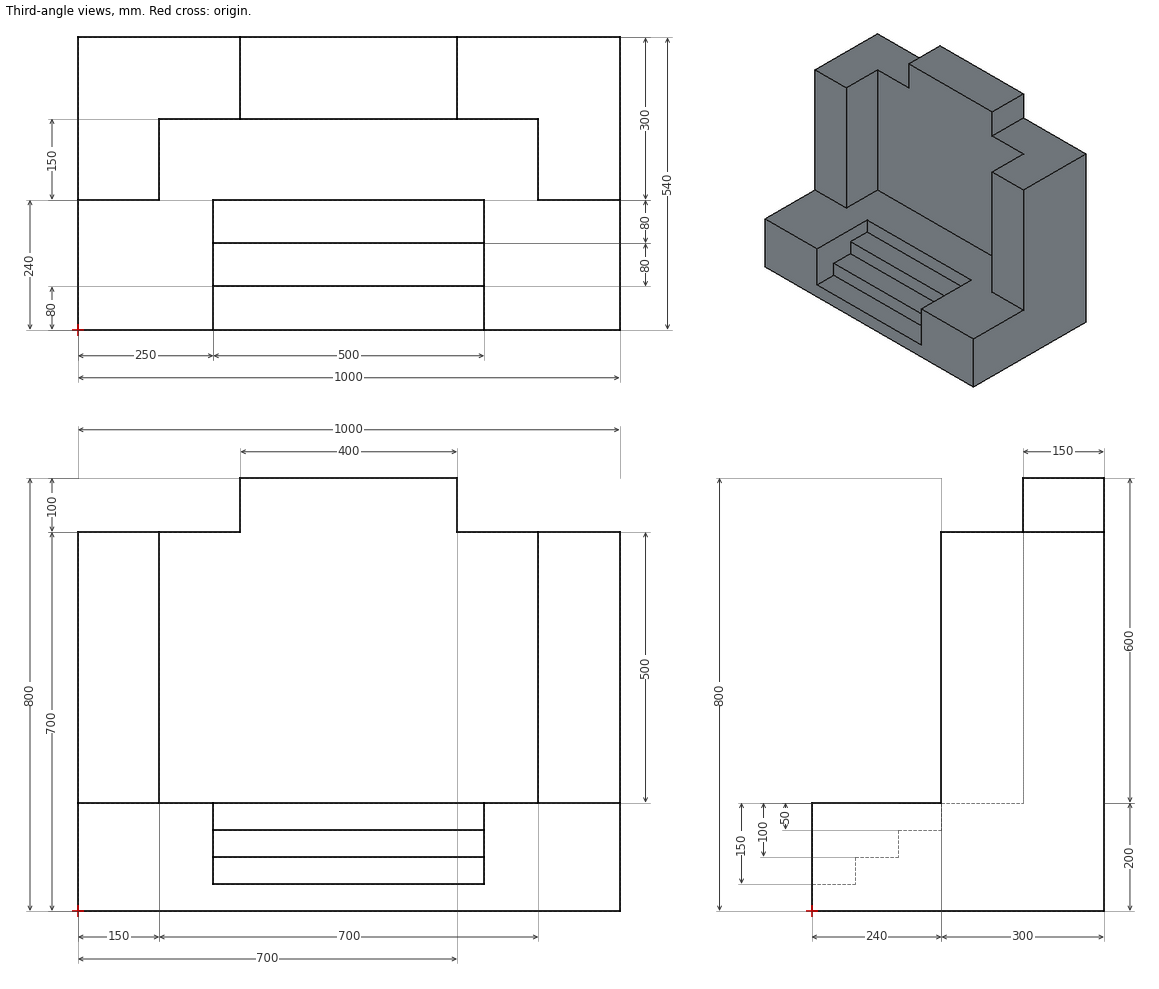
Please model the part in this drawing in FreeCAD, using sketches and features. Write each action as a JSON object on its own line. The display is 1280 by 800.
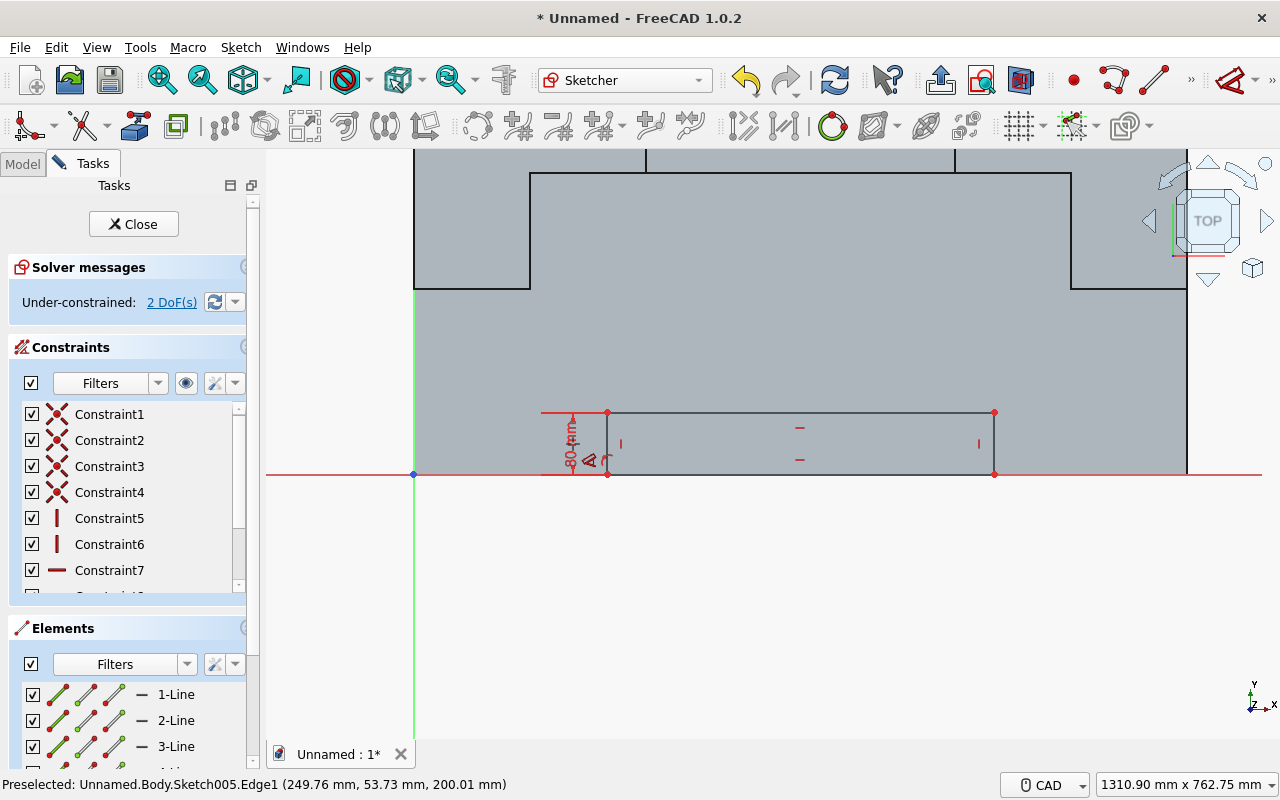
{"action": "left_click", "coordinate": [723, 475]}
{"action": "left_click", "coordinate": [801, 509]}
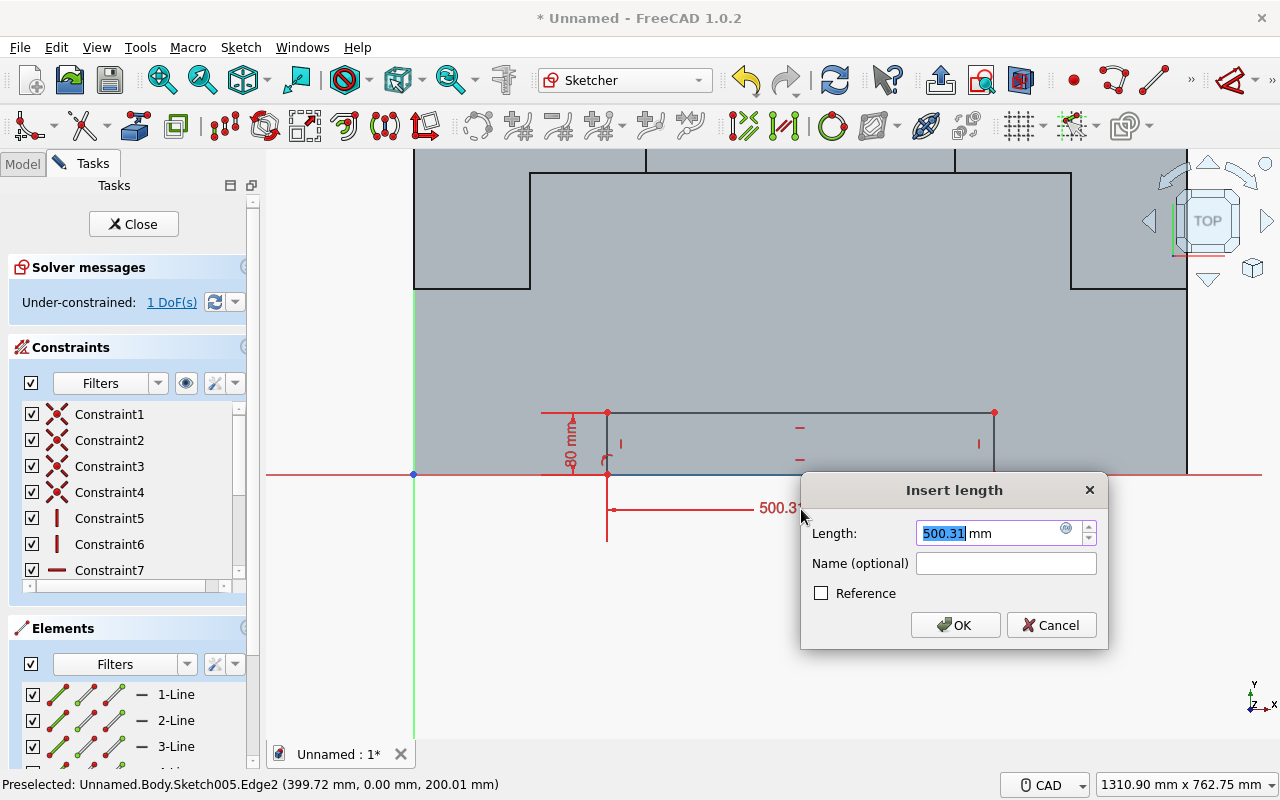
{"action": "type", "text": "500"}
{"action": "key", "text": "Return"}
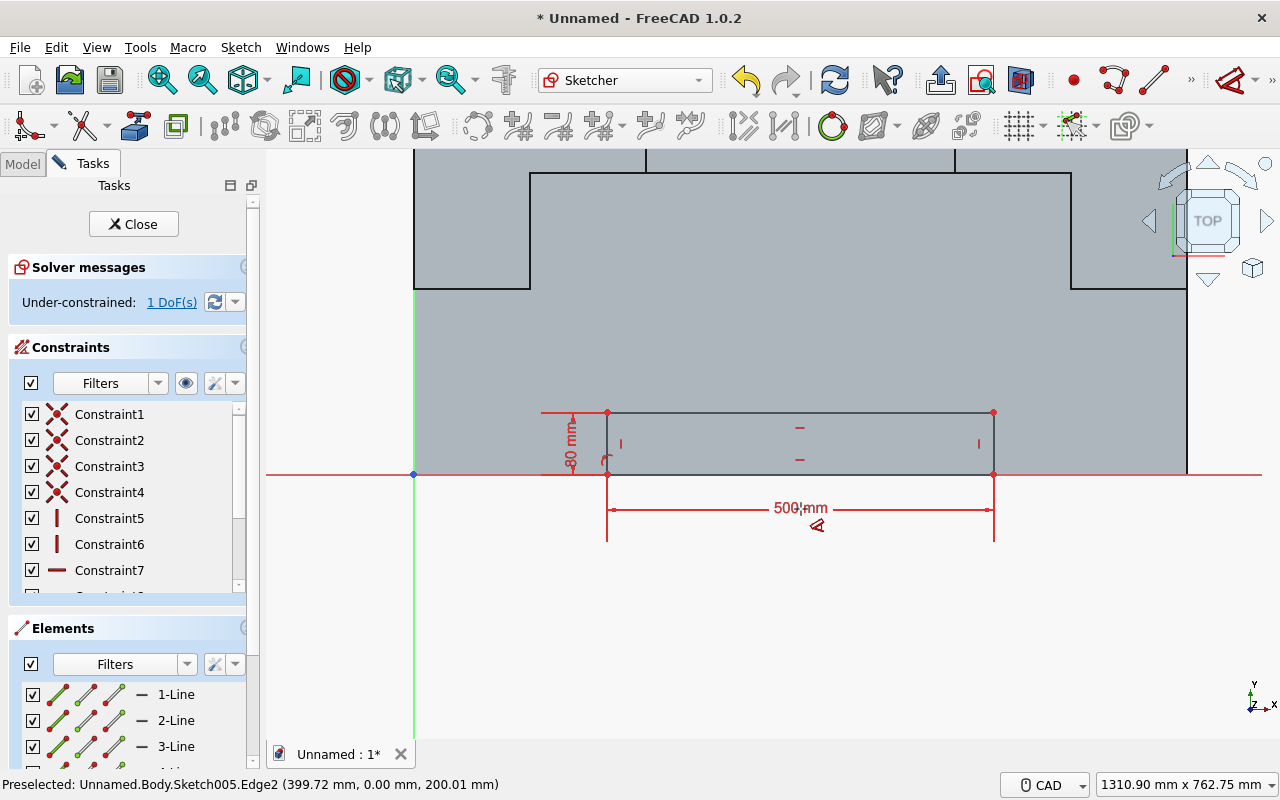
{"action": "left_click", "coordinate": [607, 413]}
{"action": "left_click", "coordinate": [510, 509]}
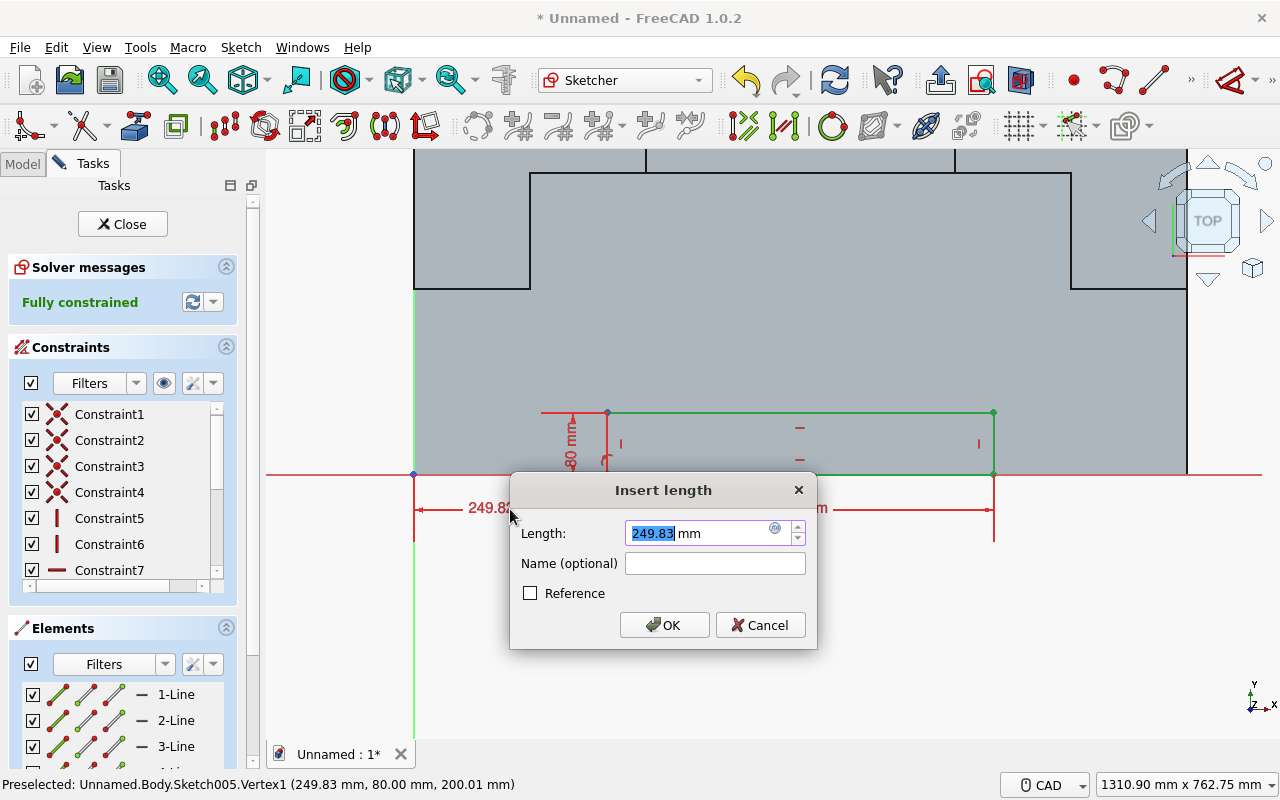
{"action": "type", "text": "250"}
{"action": "key", "text": "Return"}
{"action": "key", "text": "Escape"}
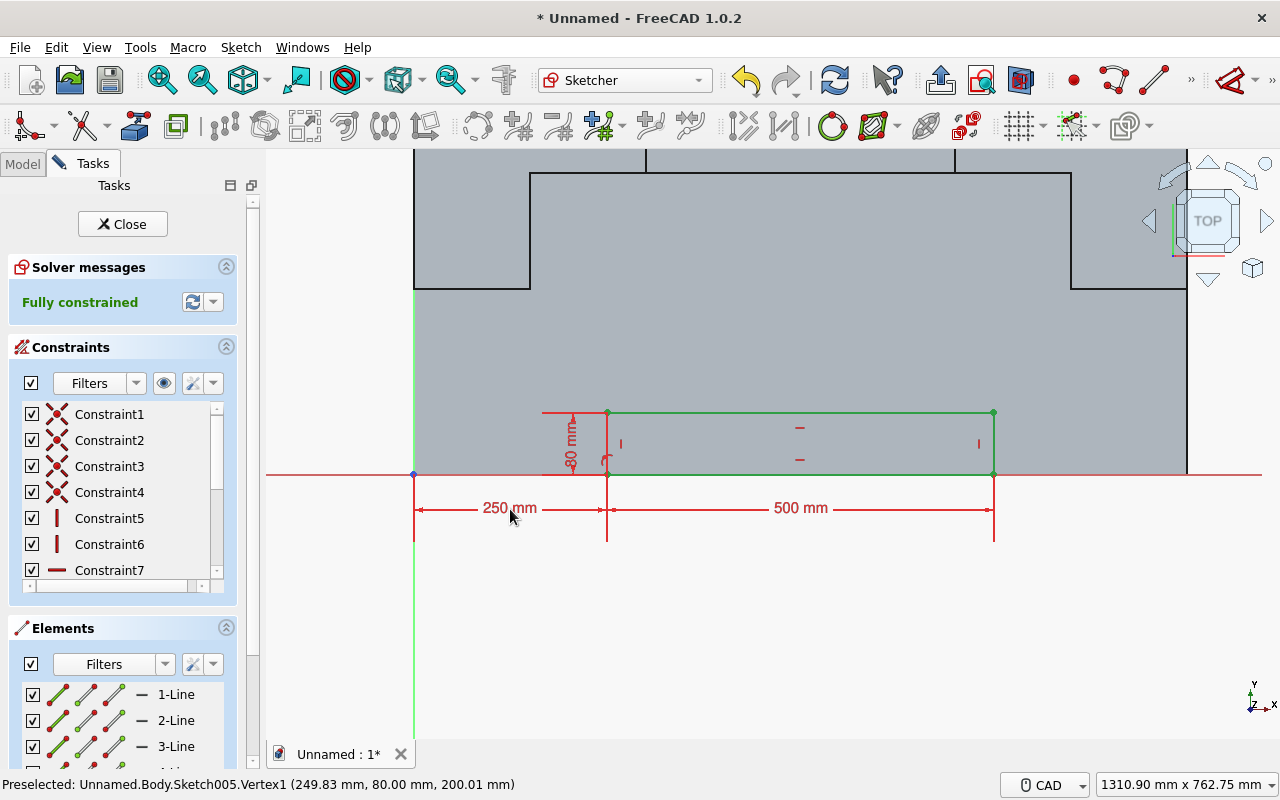
{"action": "left_click", "coordinate": [123, 224]}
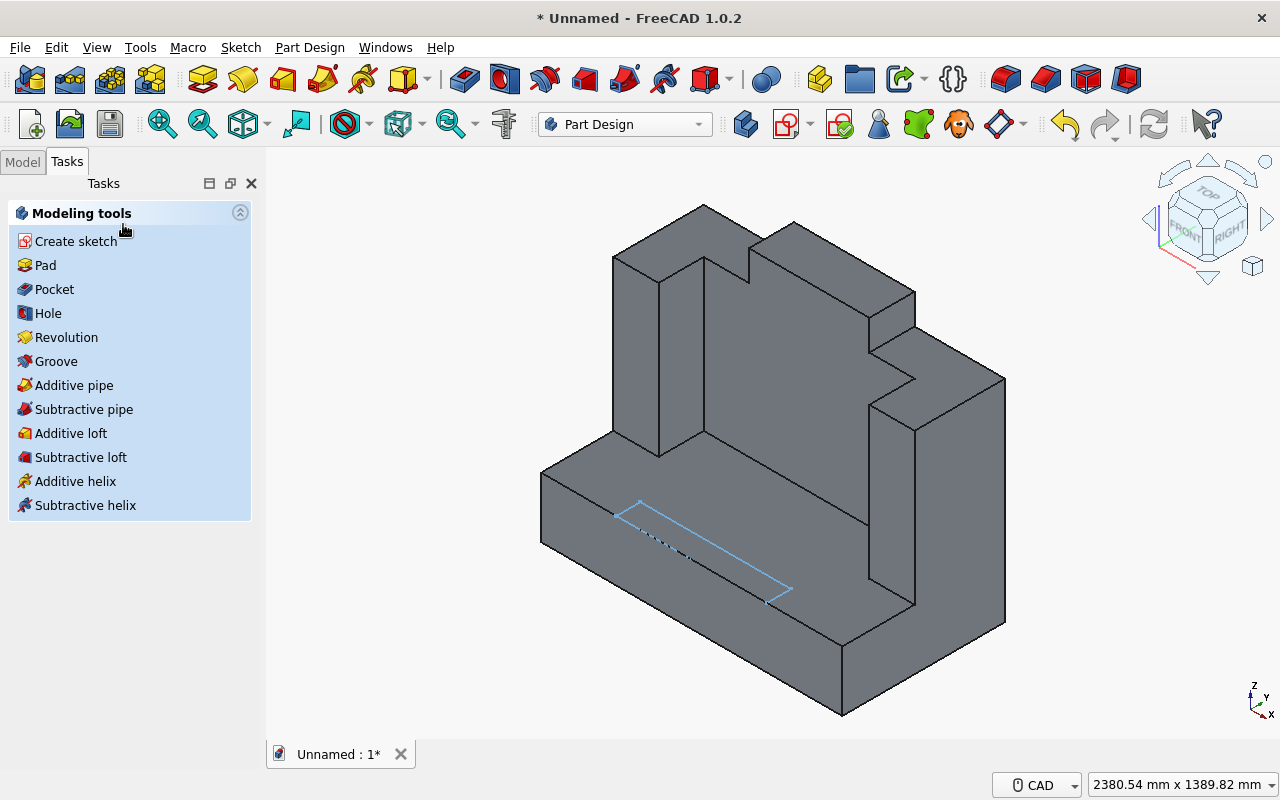
{"action": "left_click", "coordinate": [466, 80]}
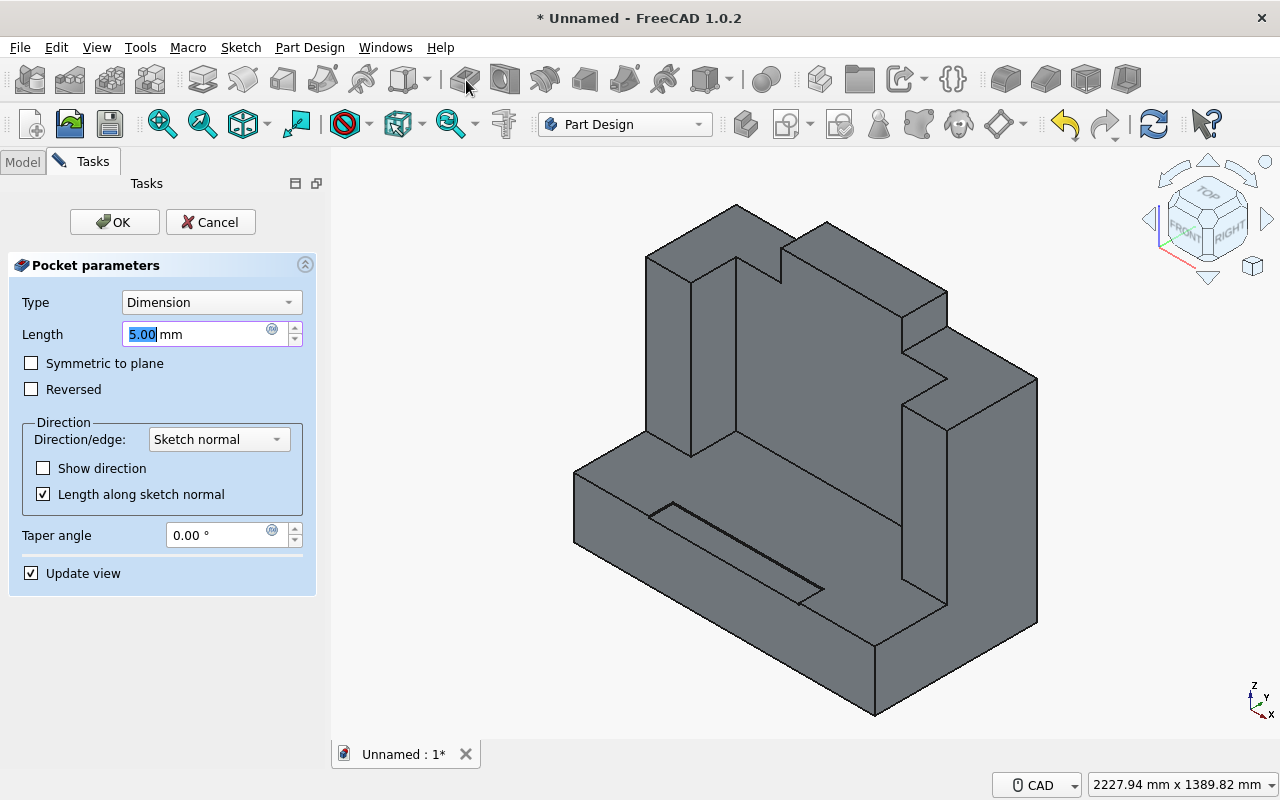
{"action": "type", "text": "150"}
{"action": "key", "text": "Tab"}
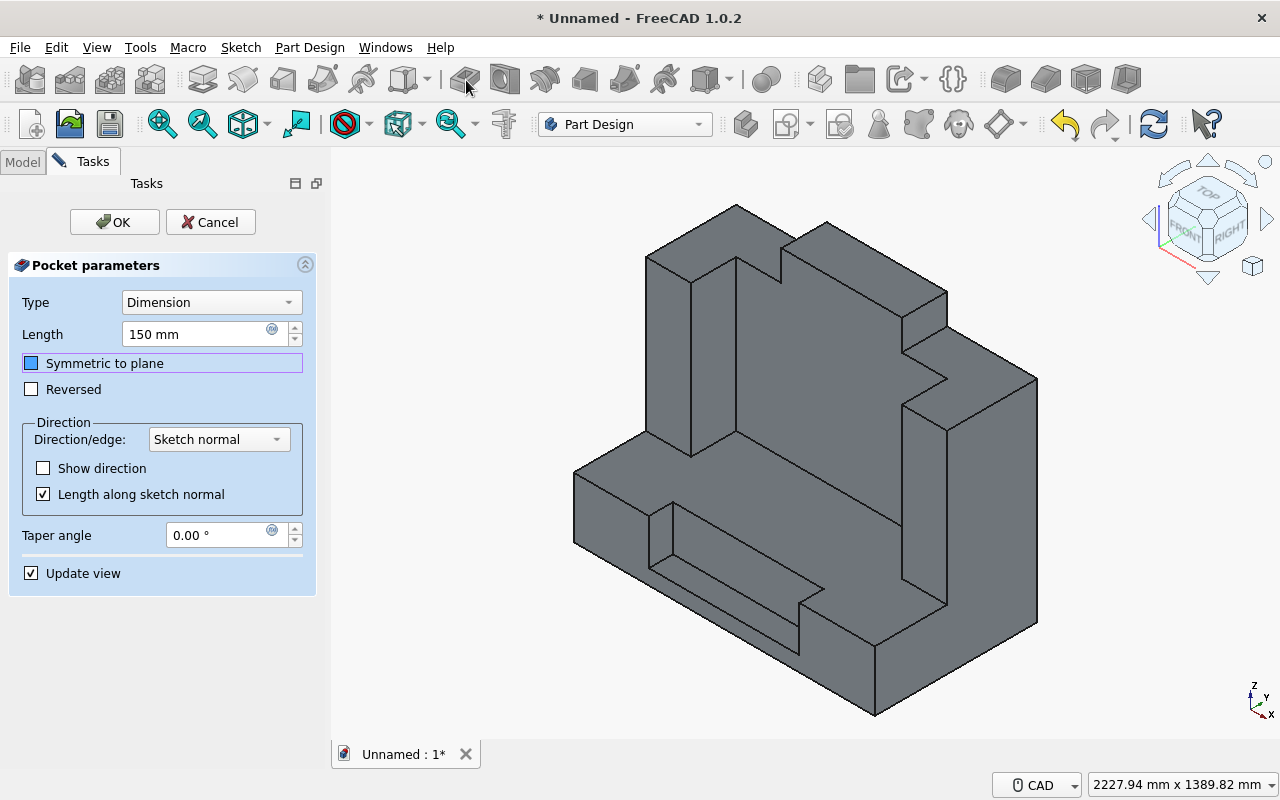
{"action": "left_click", "coordinate": [115, 222]}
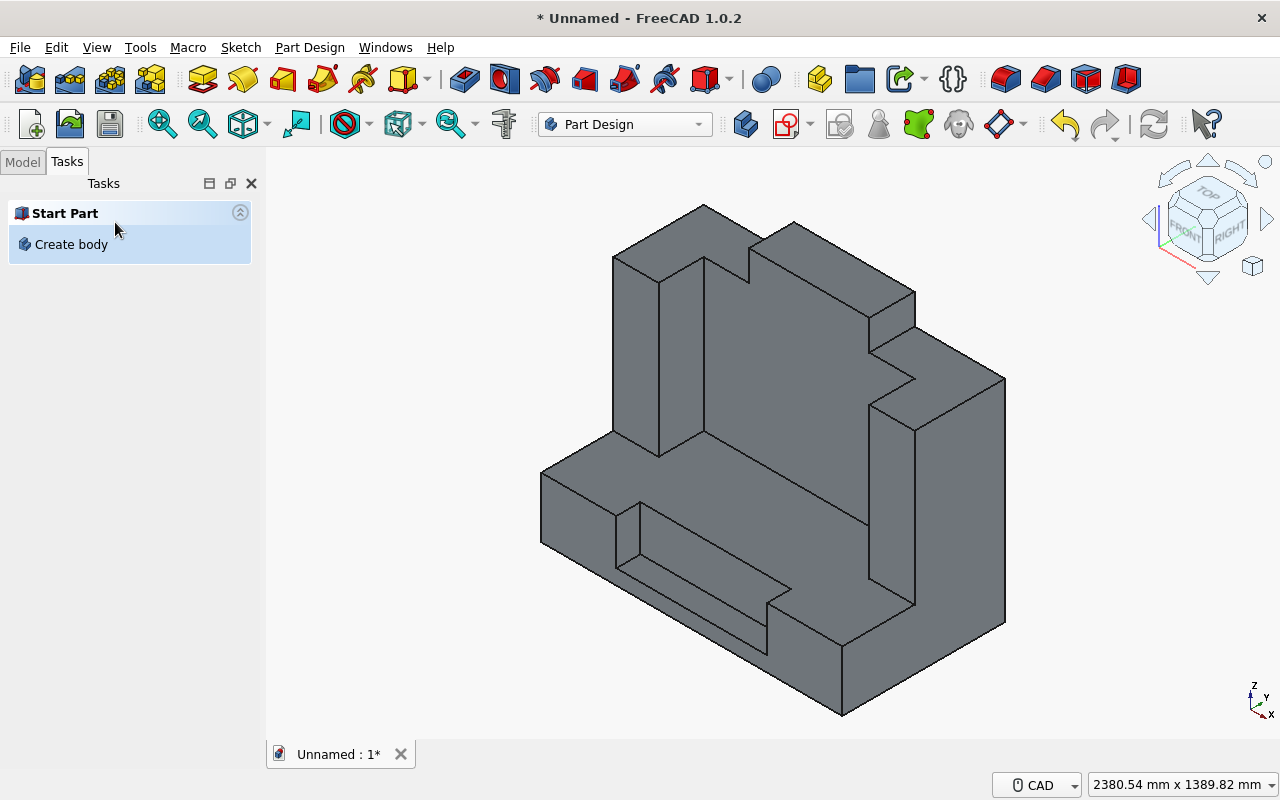
{"action": "left_click", "coordinate": [810, 540]}